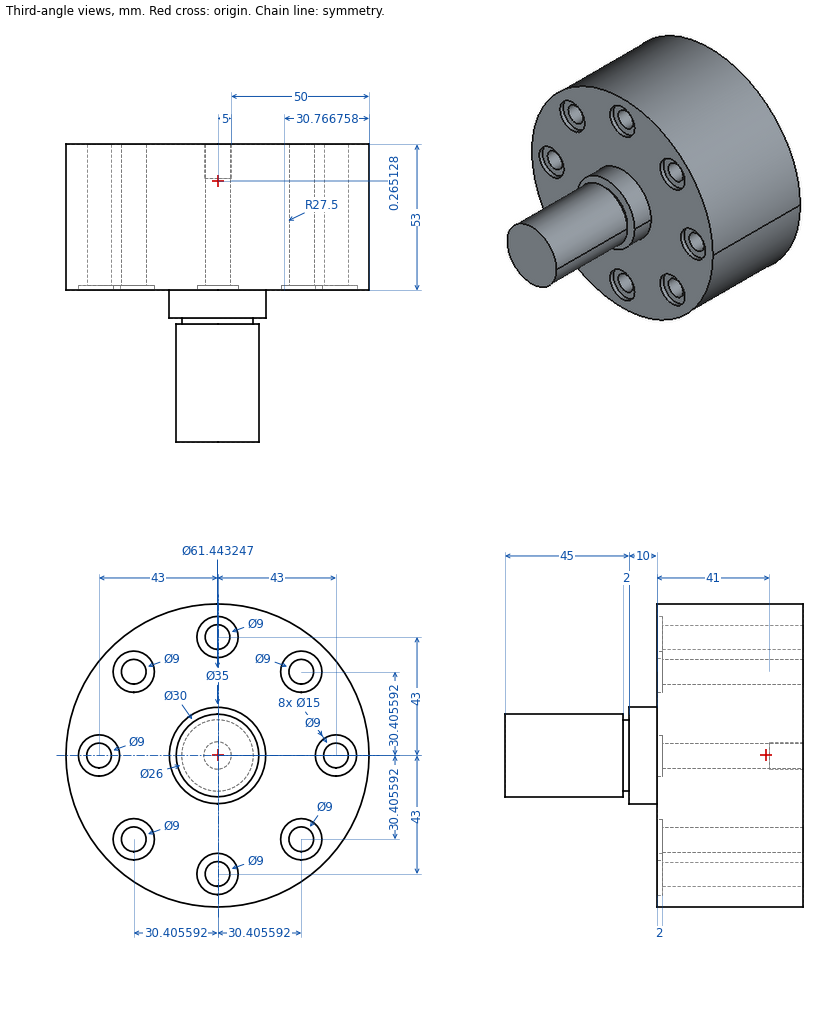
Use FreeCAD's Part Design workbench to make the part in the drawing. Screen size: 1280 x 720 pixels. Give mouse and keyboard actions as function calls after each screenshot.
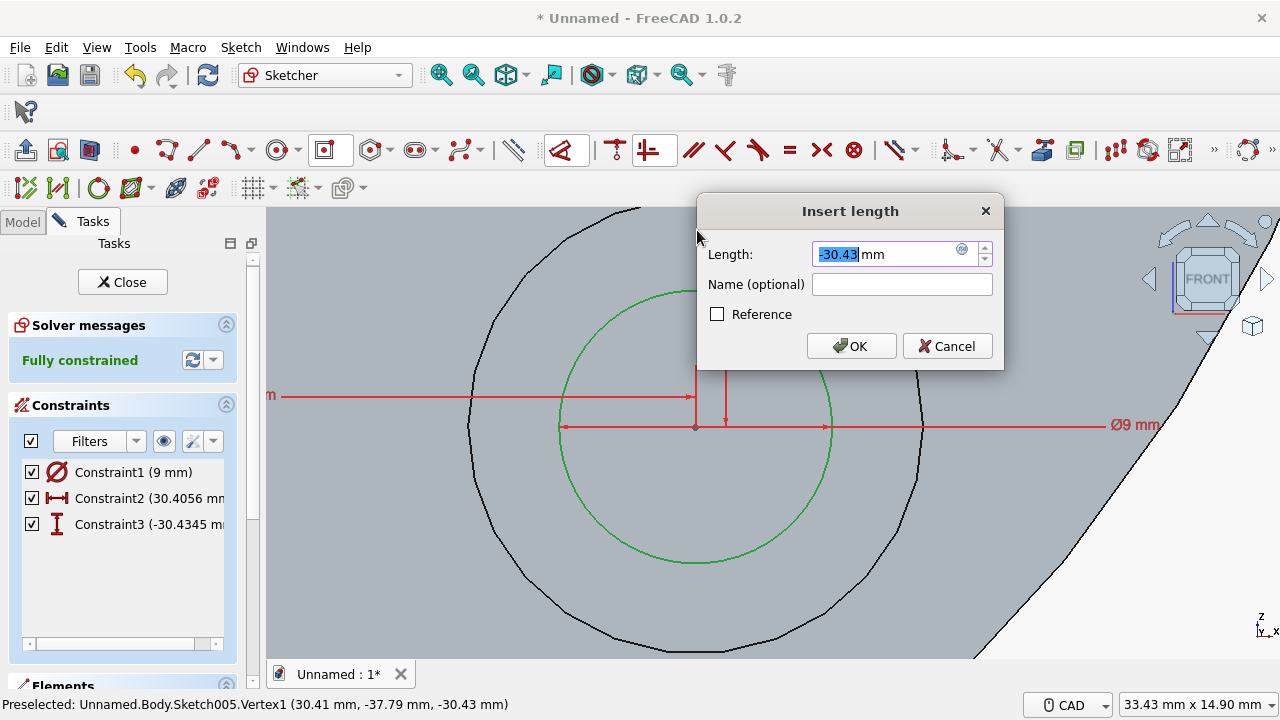
text(-30.405592)
key(Return)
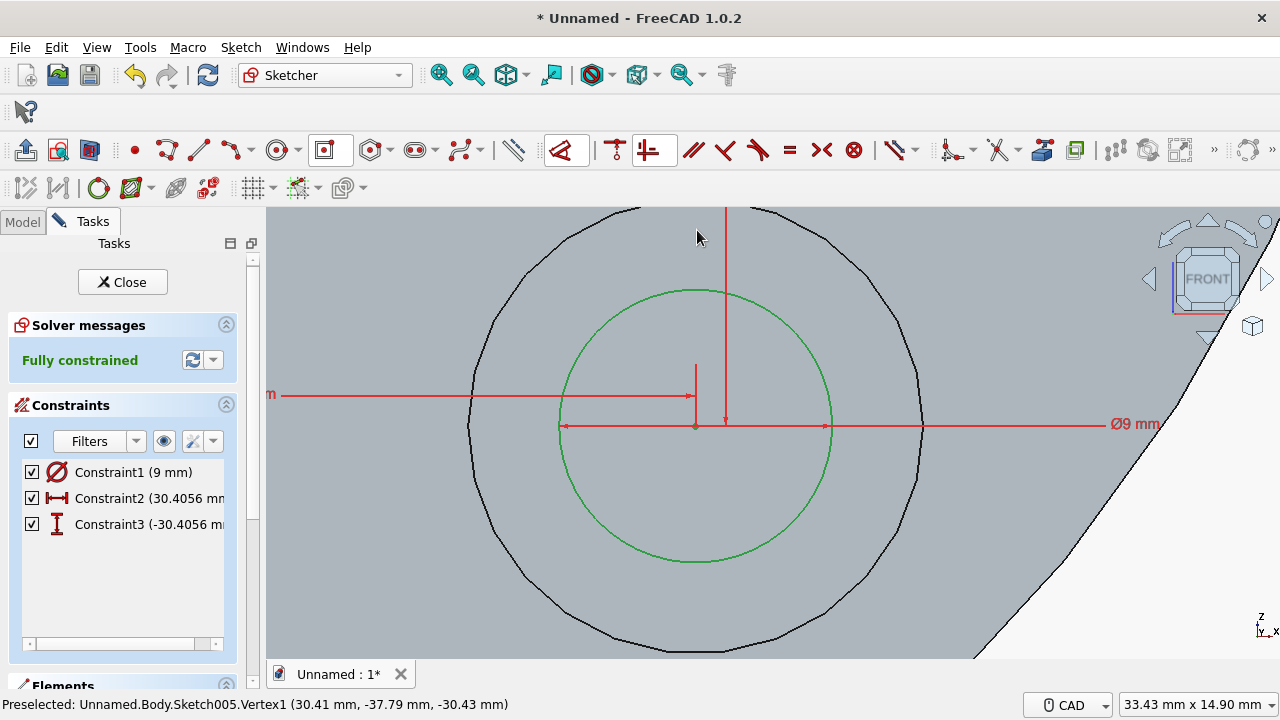
click(123, 282)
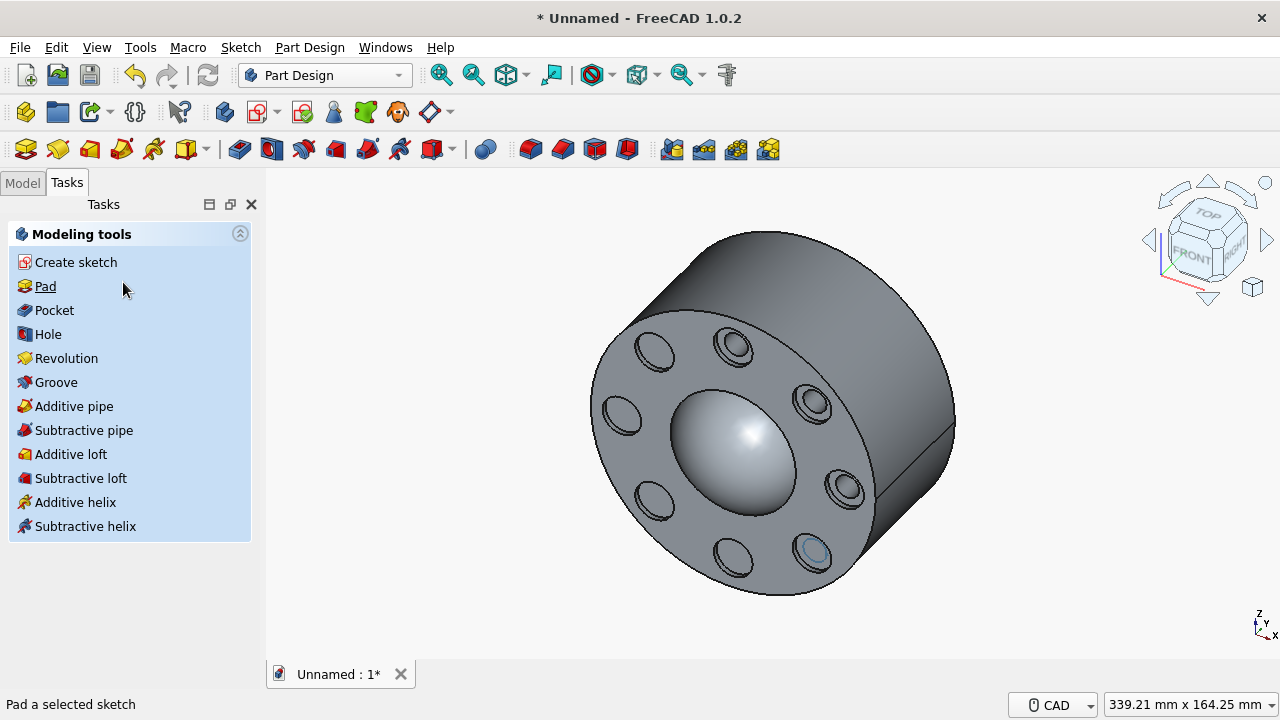
click(240, 150)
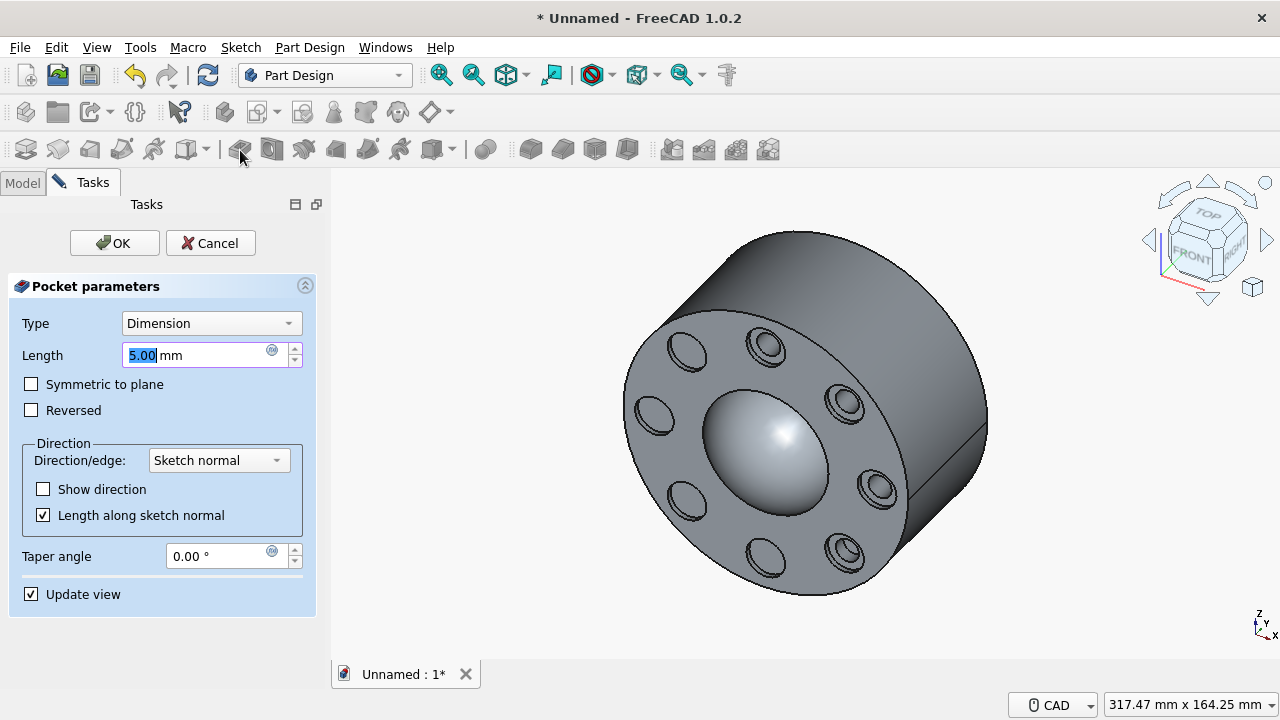
click(212, 324)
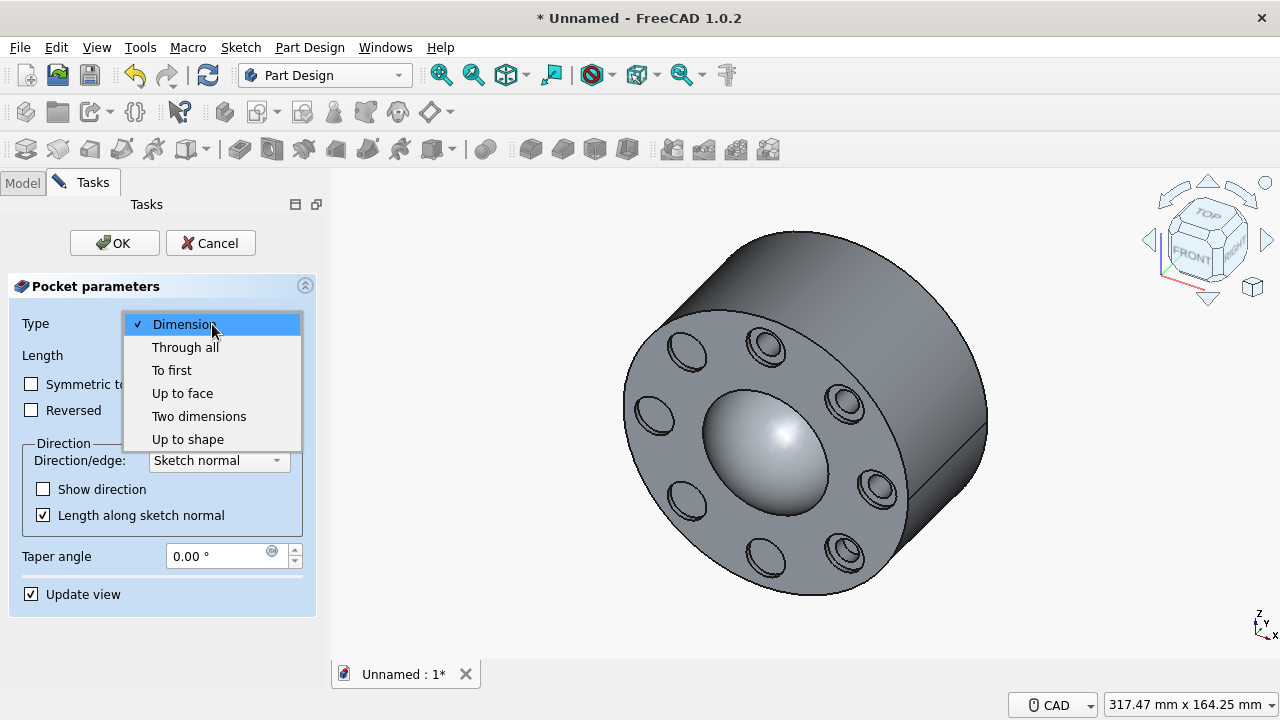
click(212, 370)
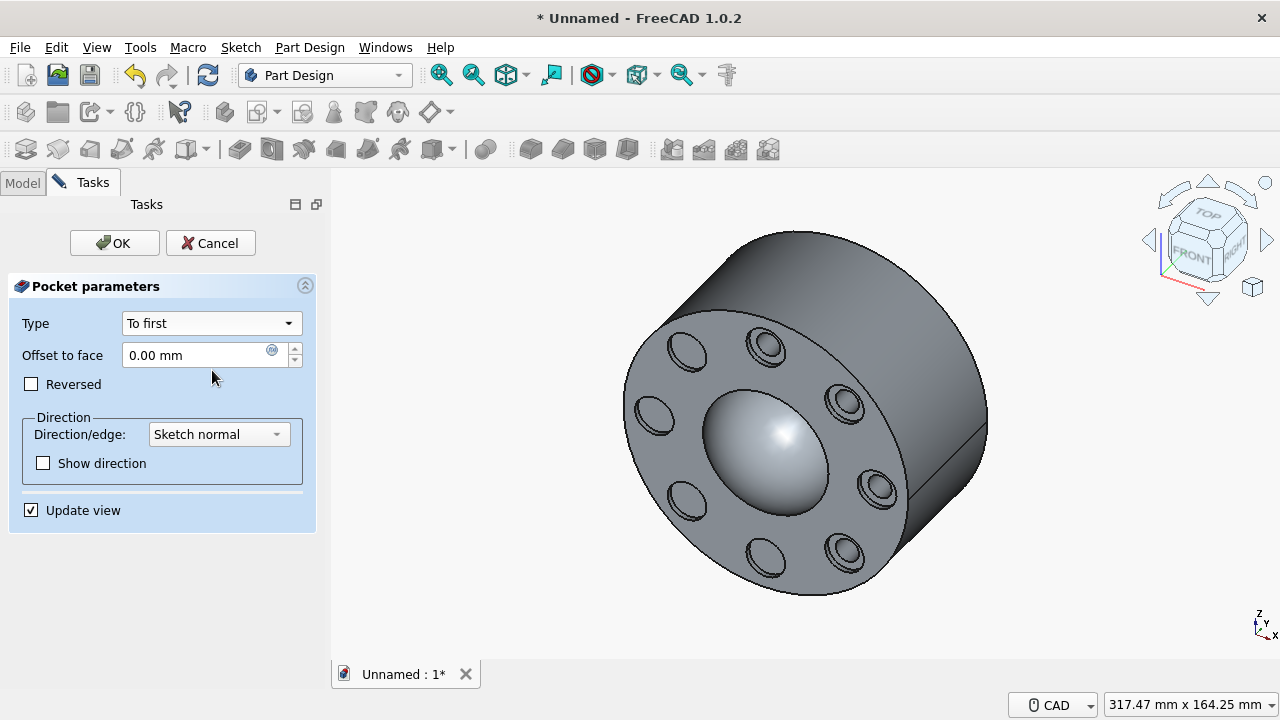
click(115, 243)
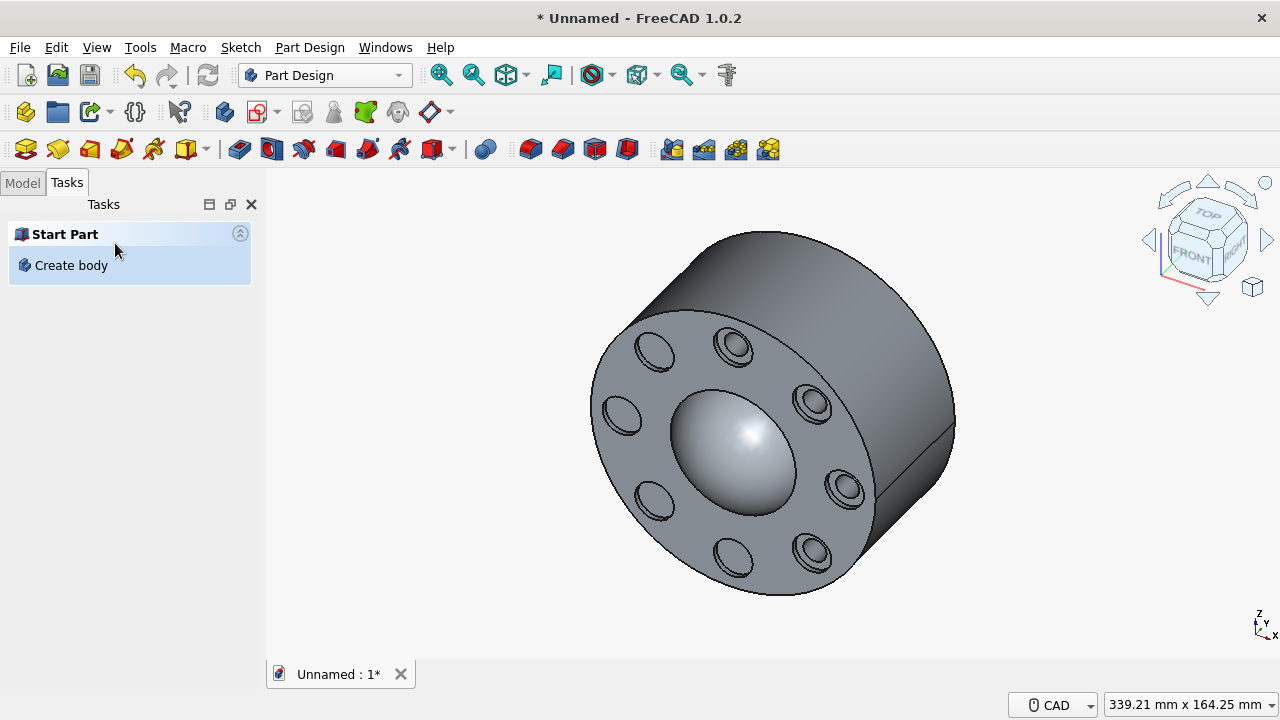
click(658, 348)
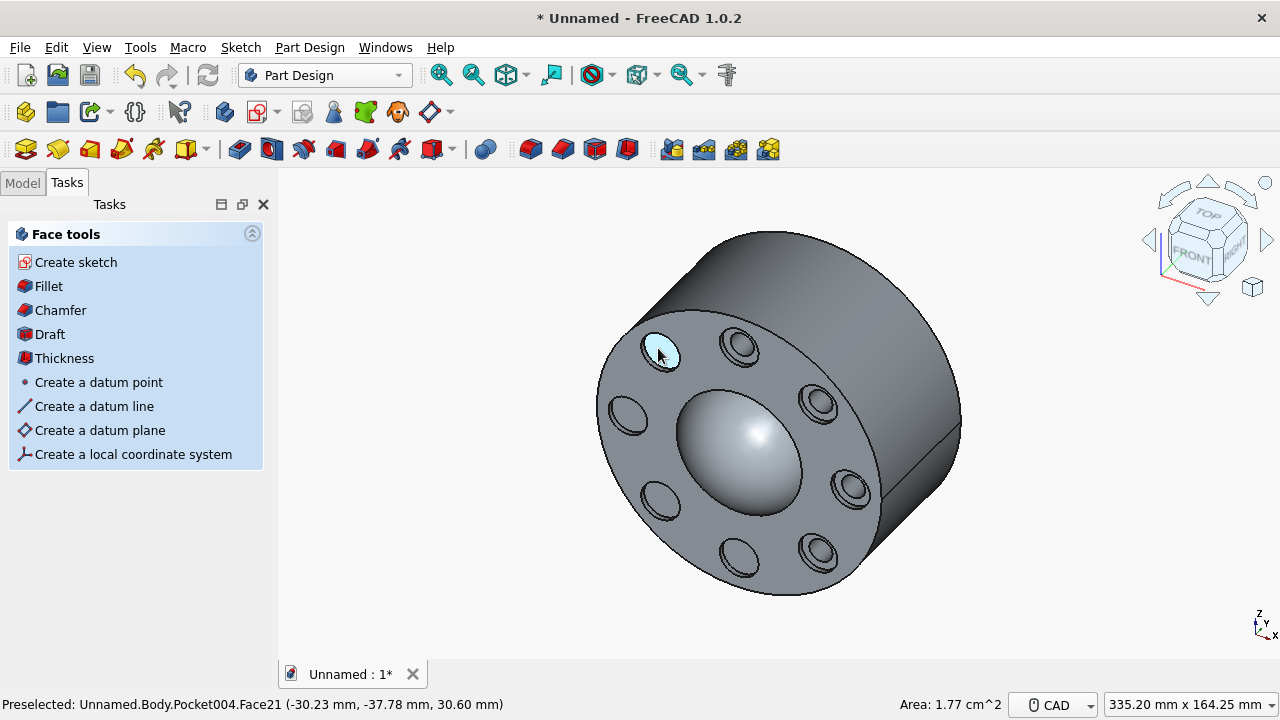
click(258, 112)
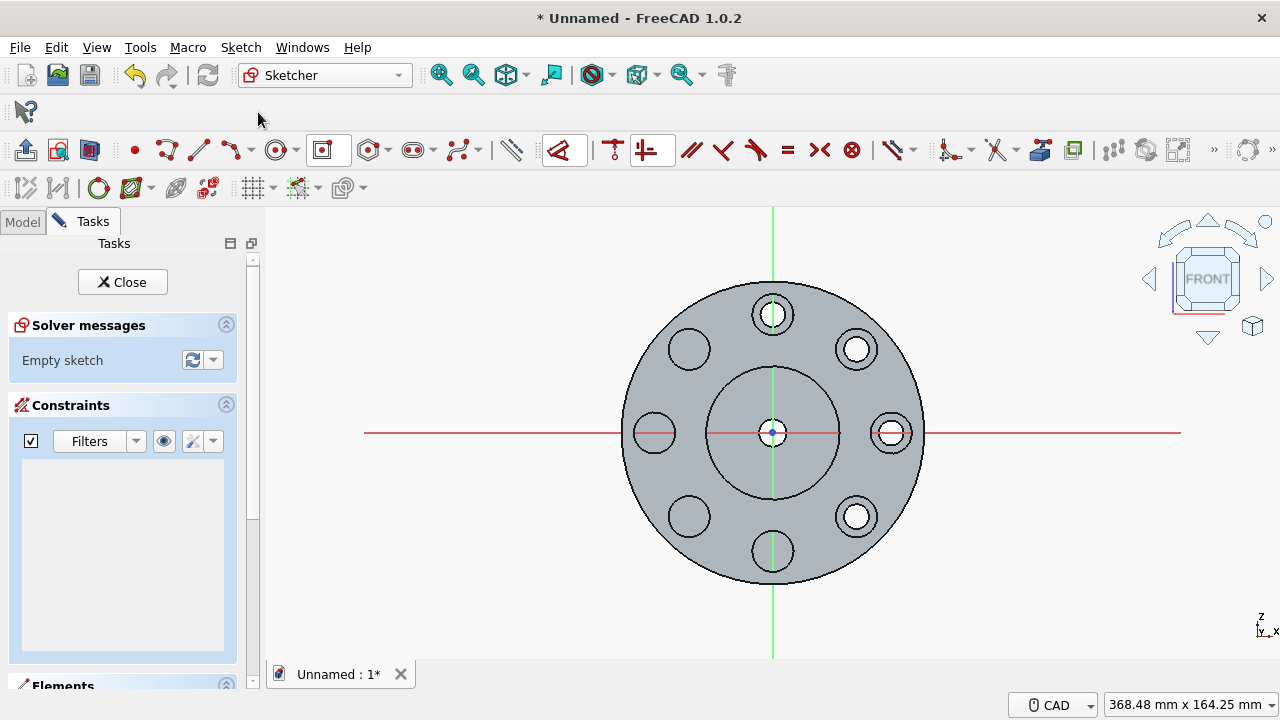
click(90, 150)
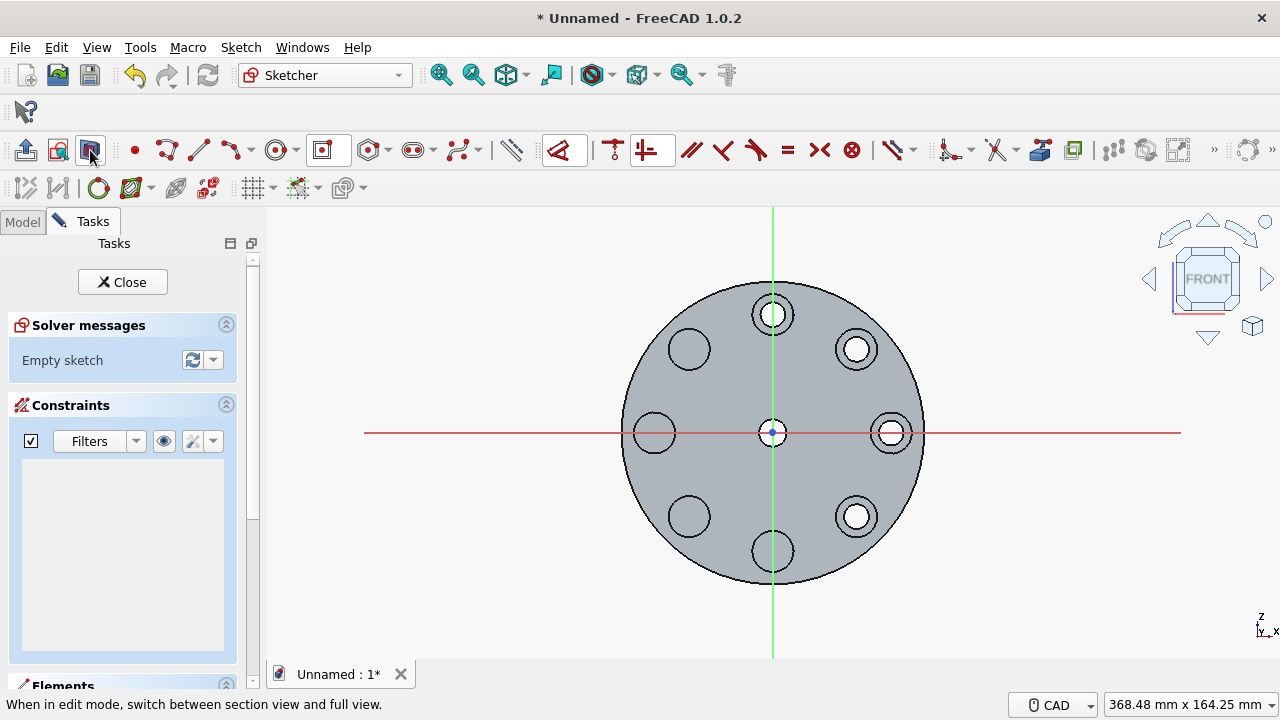
scroll(780, 563, up, 12)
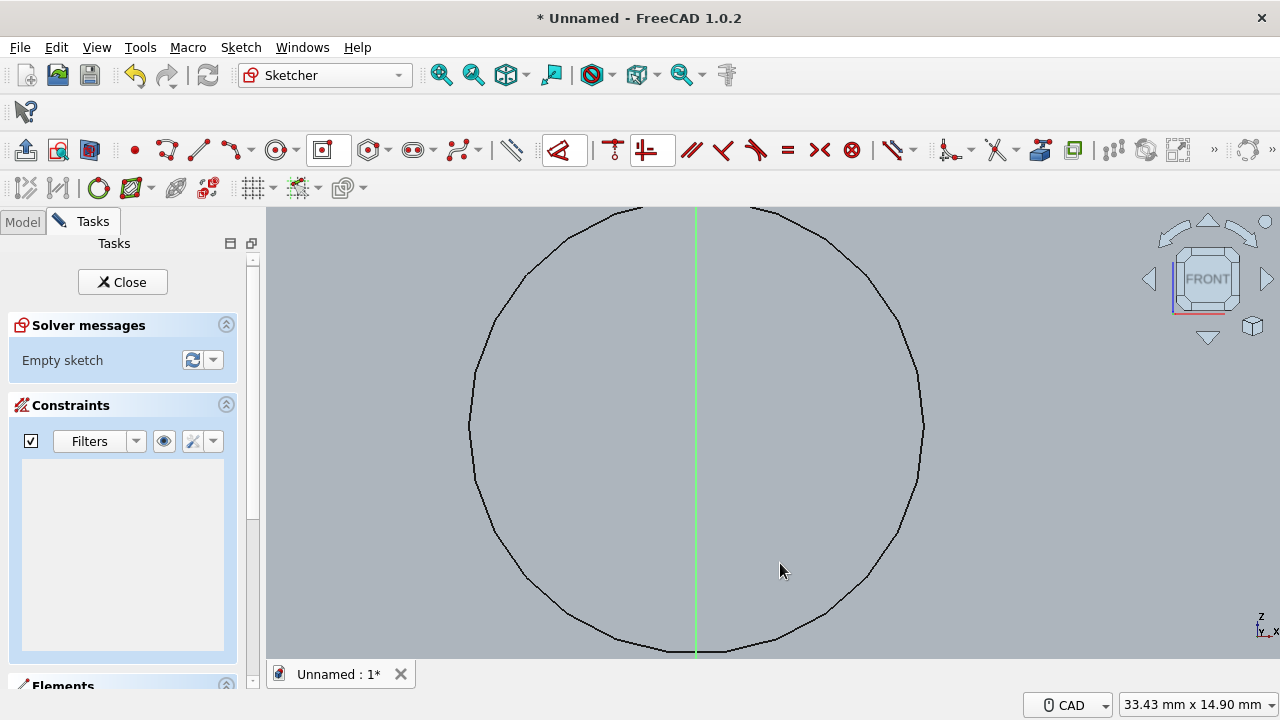
click(276, 150)